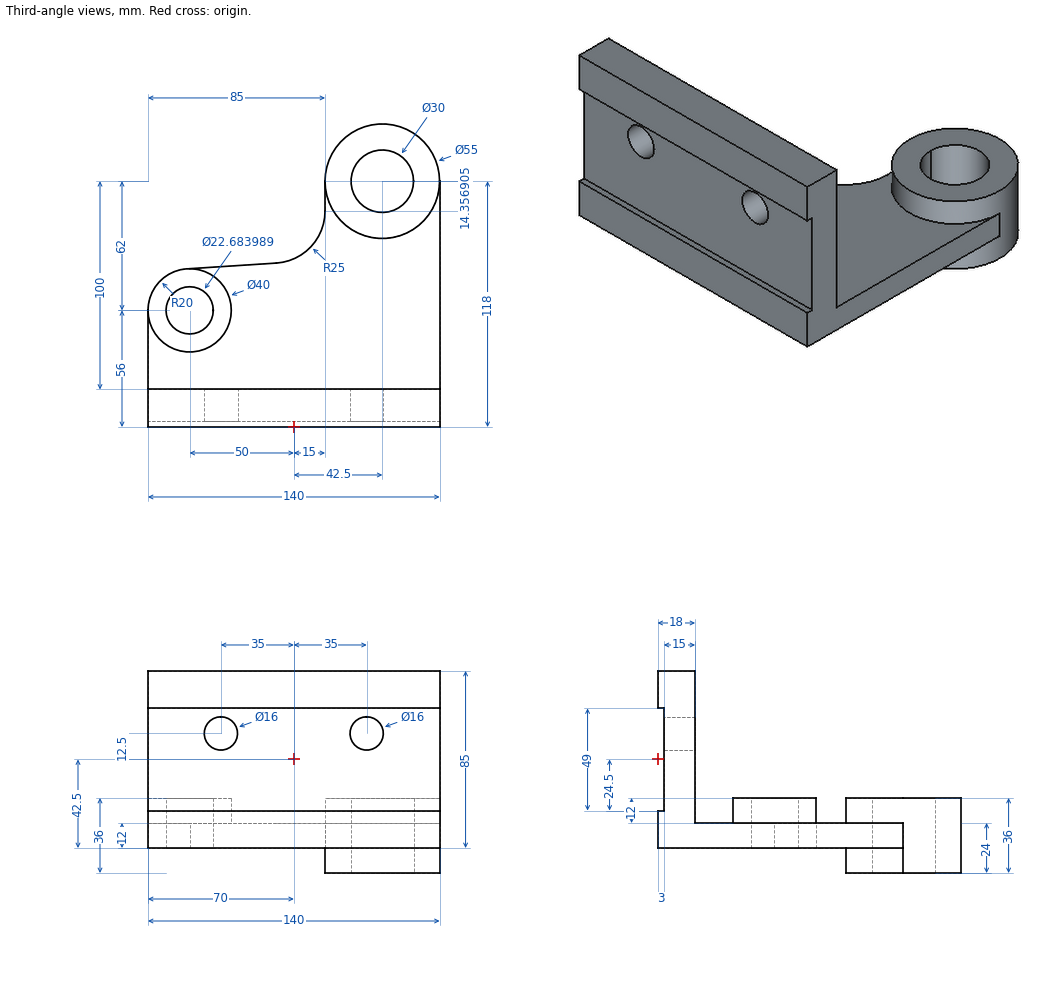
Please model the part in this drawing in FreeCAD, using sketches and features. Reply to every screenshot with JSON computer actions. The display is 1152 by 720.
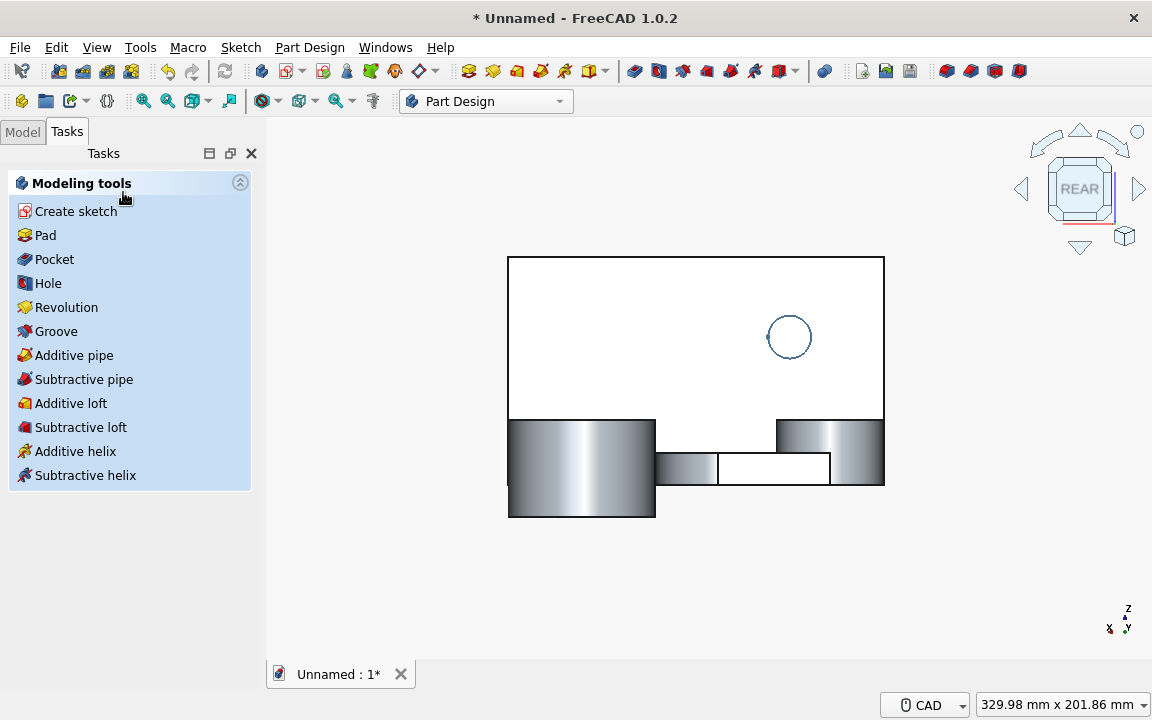
{"action": "left_click", "coordinate": [636, 72]}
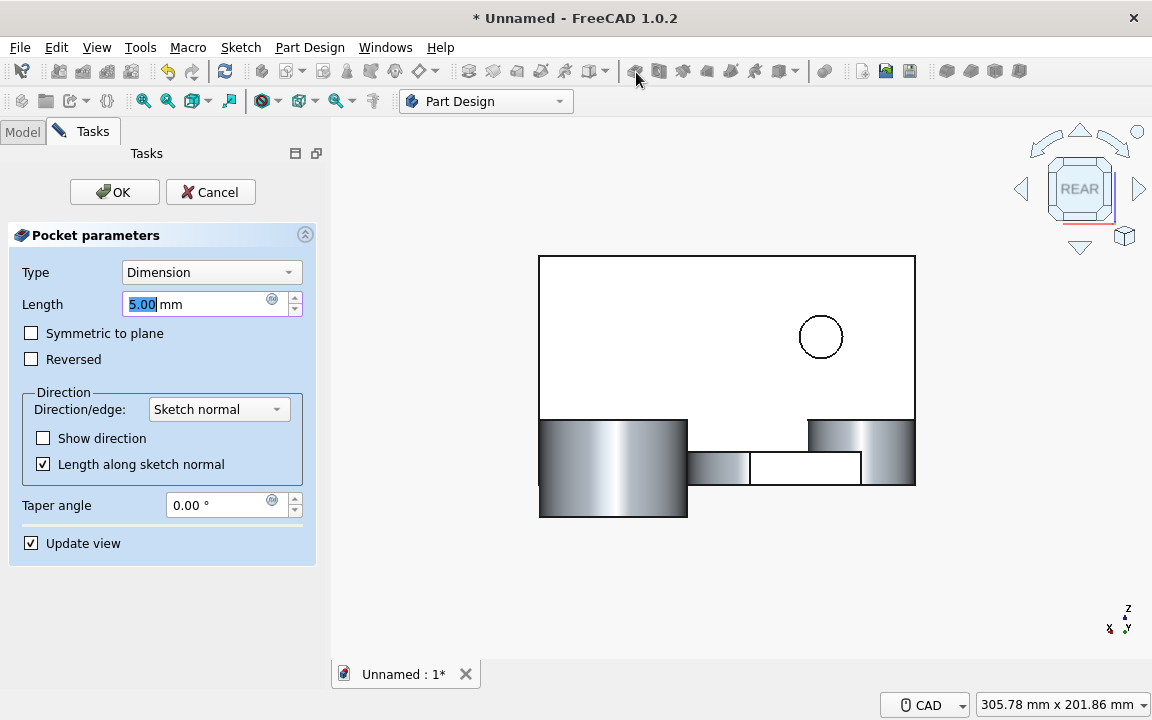
{"action": "type", "text": "15"}
{"action": "key", "text": "Tab"}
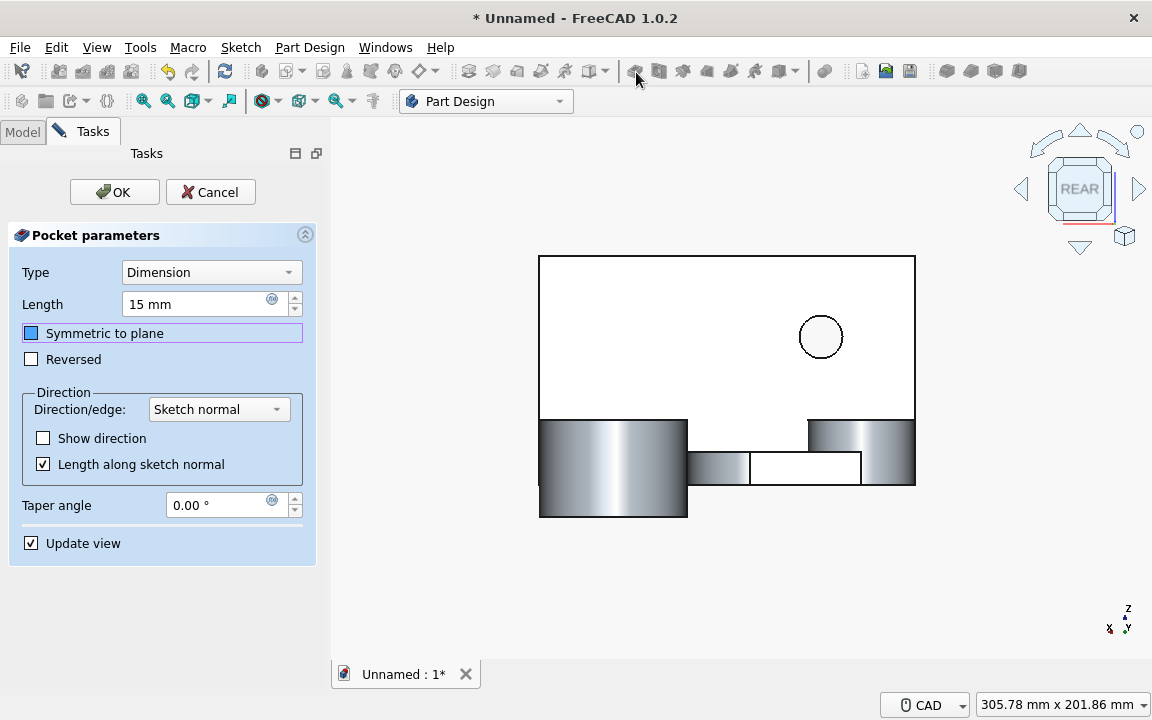
{"action": "left_click", "coordinate": [115, 192]}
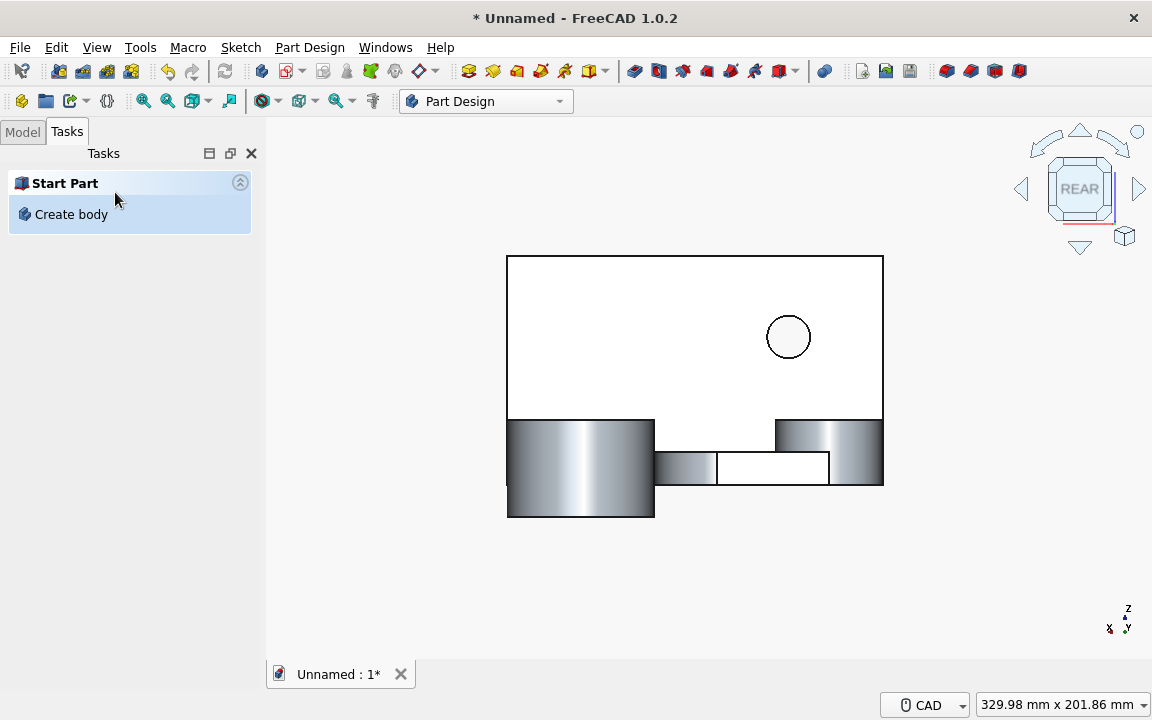
{"action": "left_click", "coordinate": [641, 353]}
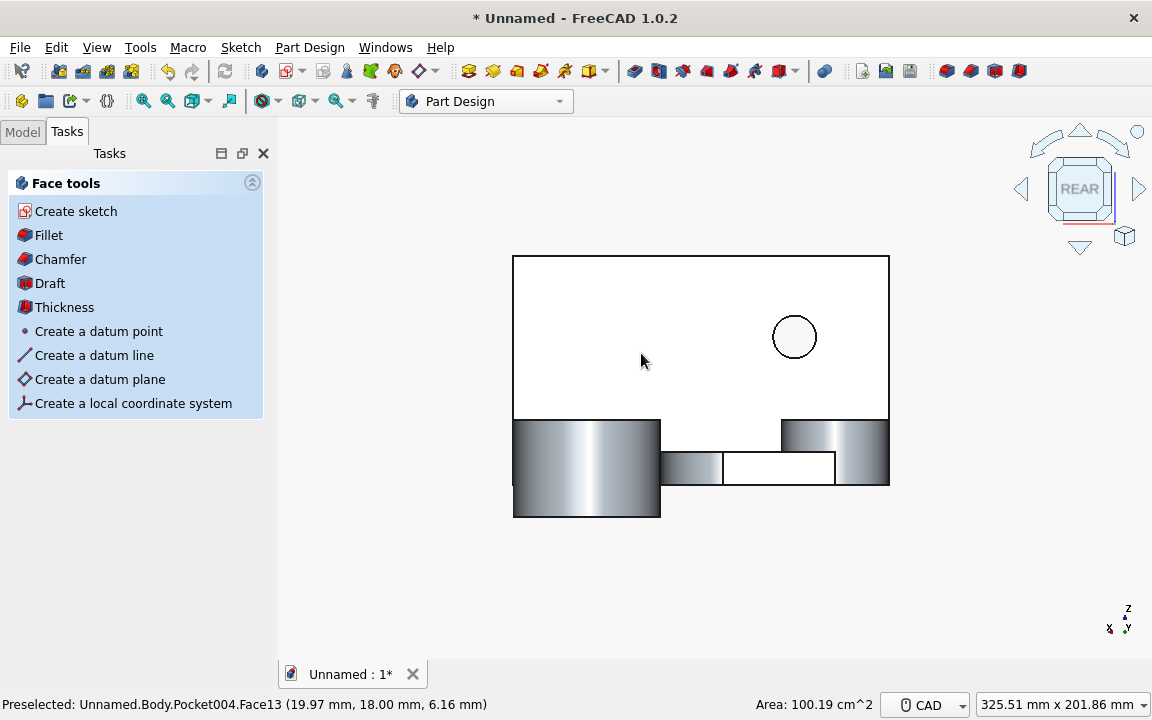
{"action": "left_click", "coordinate": [286, 72]}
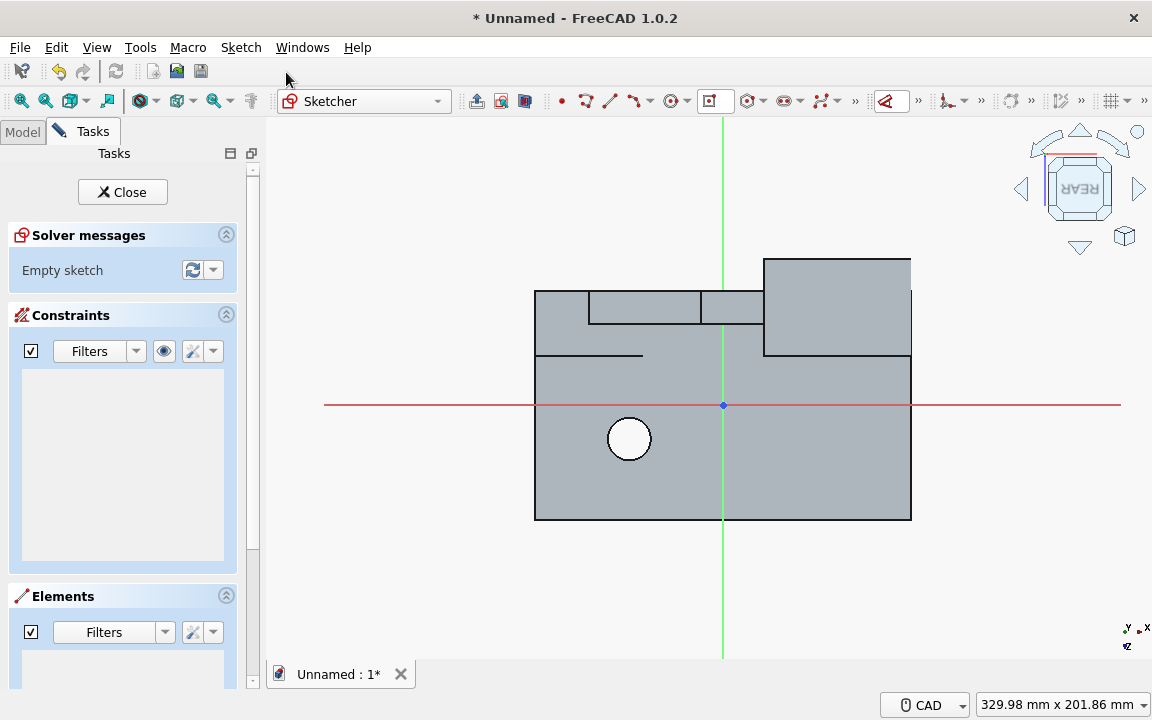
{"action": "key", "text": "q s"}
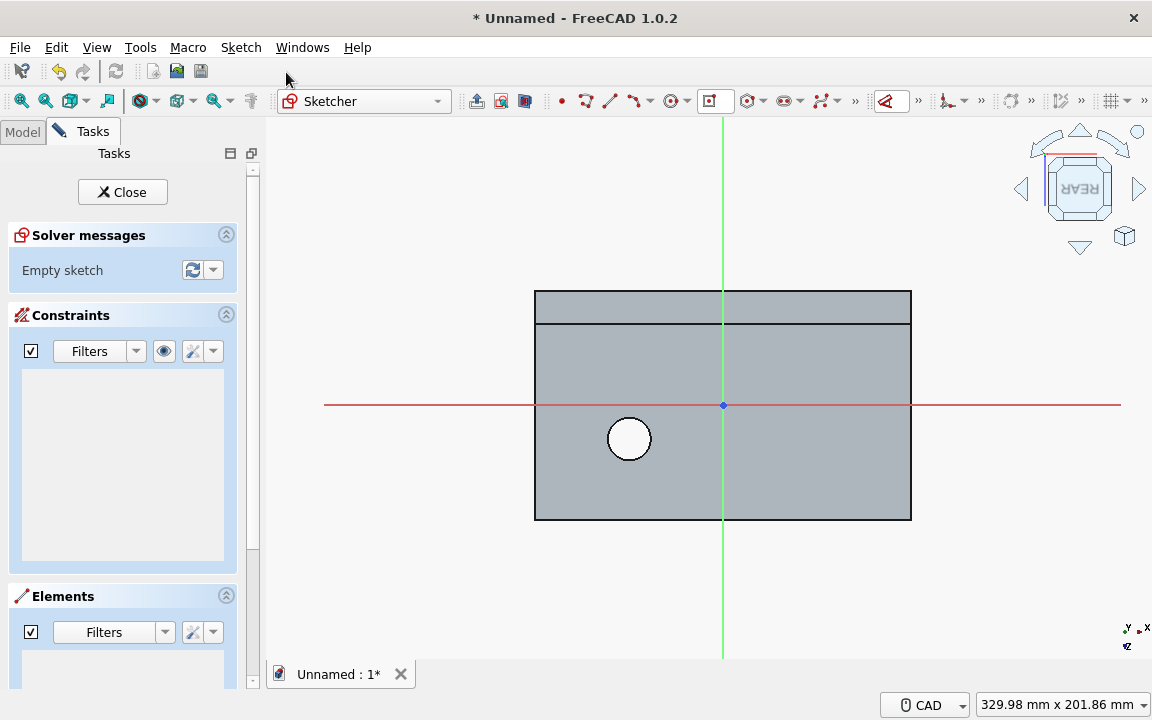
{"action": "scroll", "coordinate": [845, 447], "scroll_direction": "up", "scroll_amount": 10}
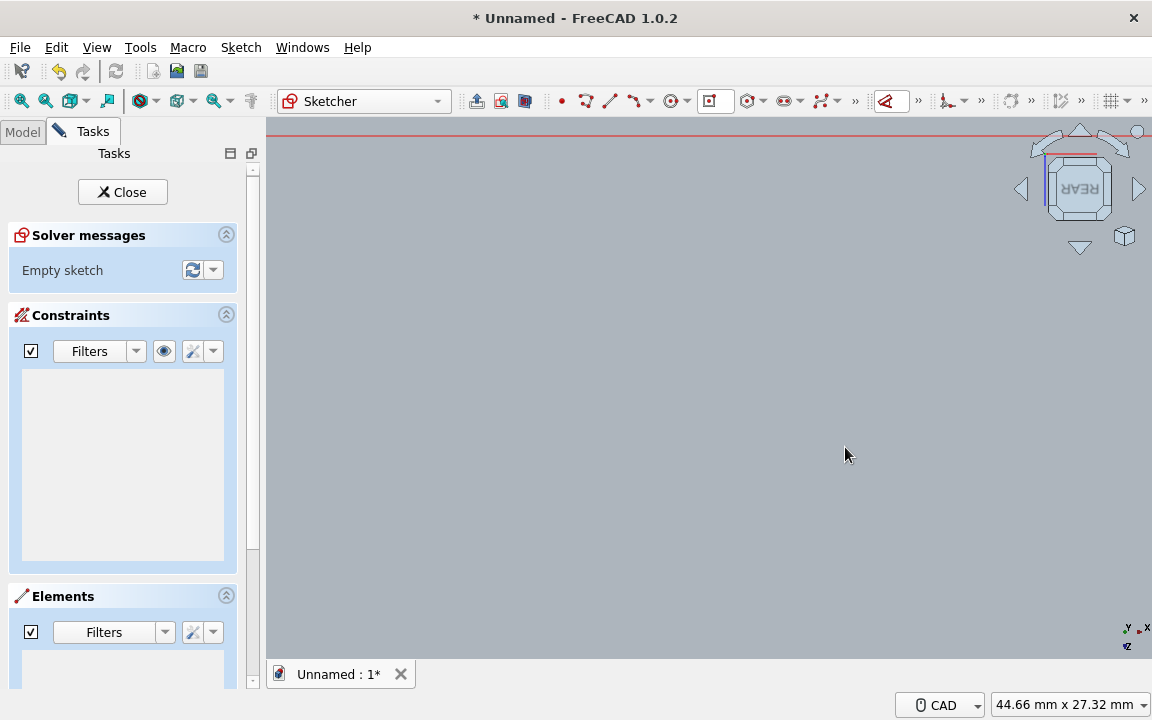
{"action": "key", "text": "g c"}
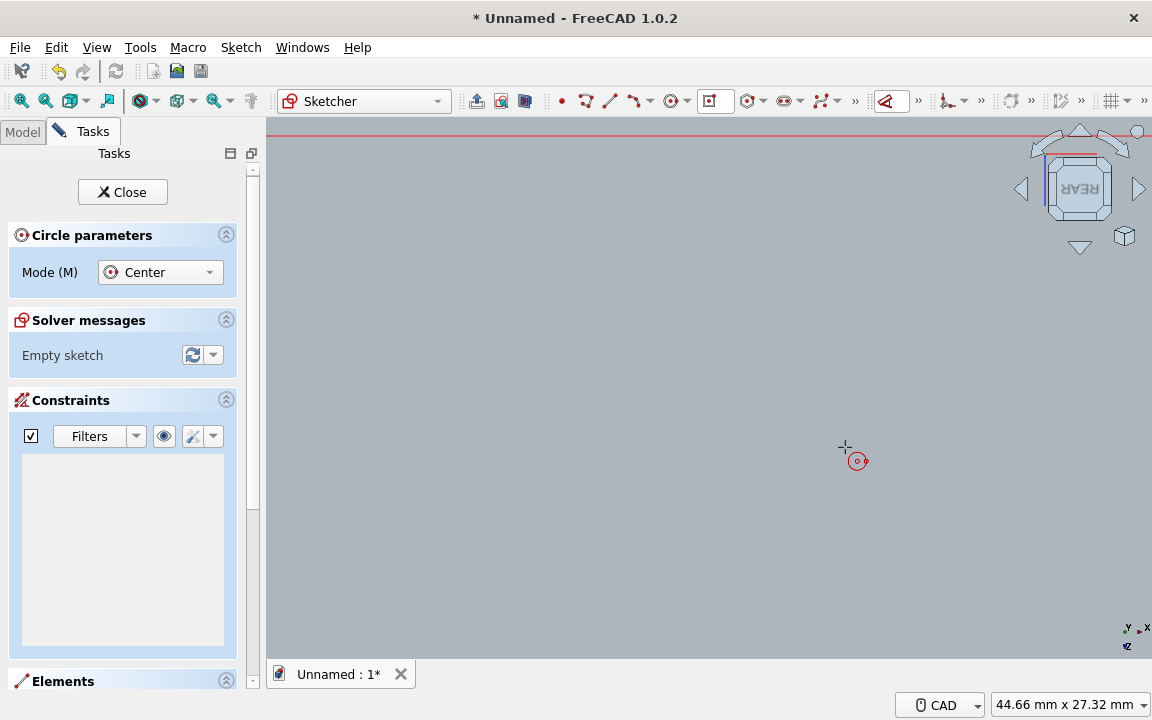
{"action": "left_click", "coordinate": [637, 384]}
{"action": "left_click", "coordinate": [749, 272]}
{"action": "key", "text": "Escape"}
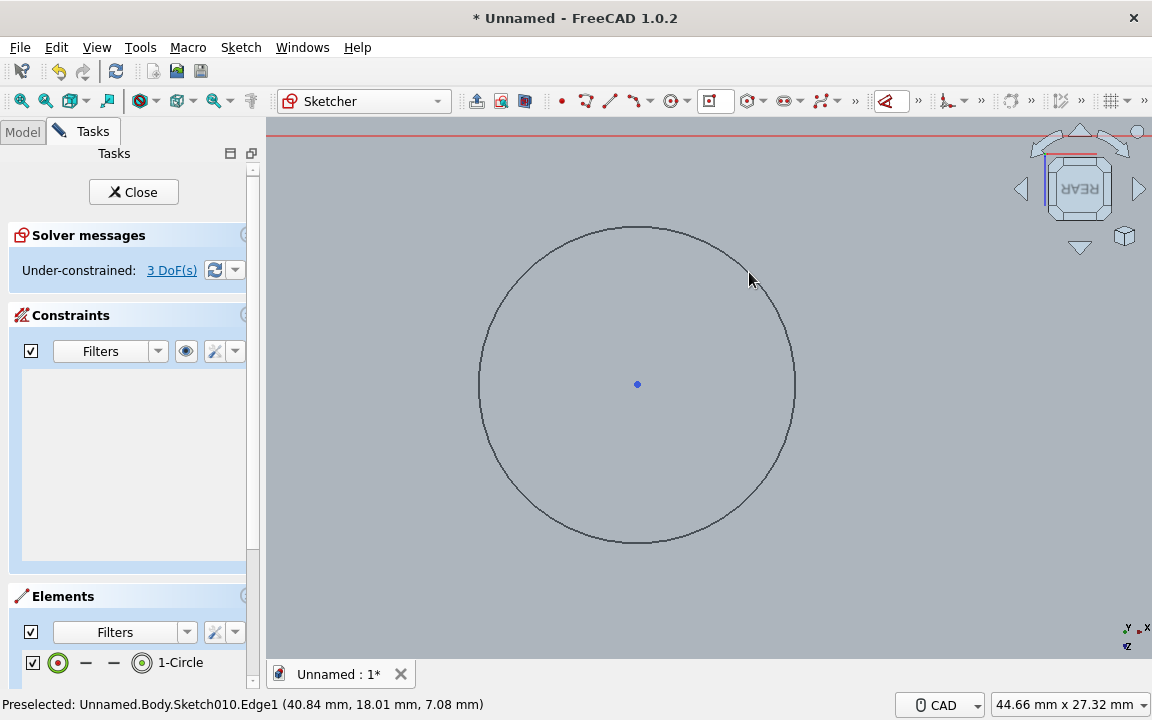
{"action": "left_click", "coordinate": [749, 273]}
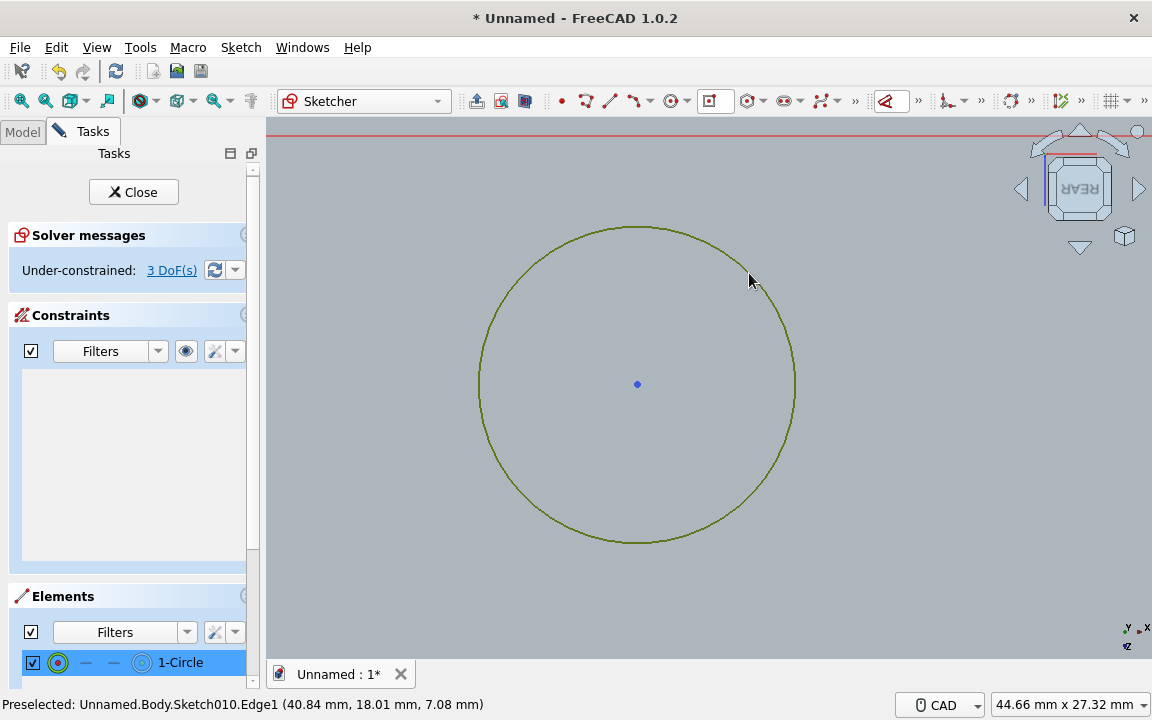
{"action": "key", "text": "k o"}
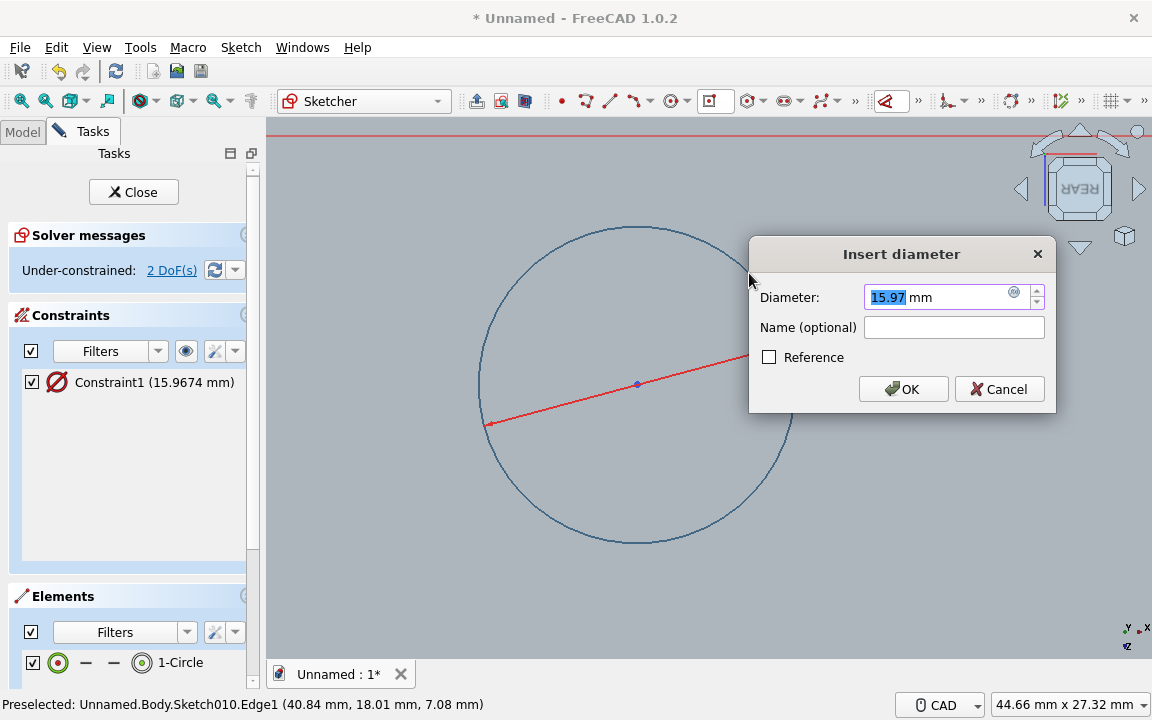
{"action": "type", "text": "16"}
{"action": "key", "text": "Return"}